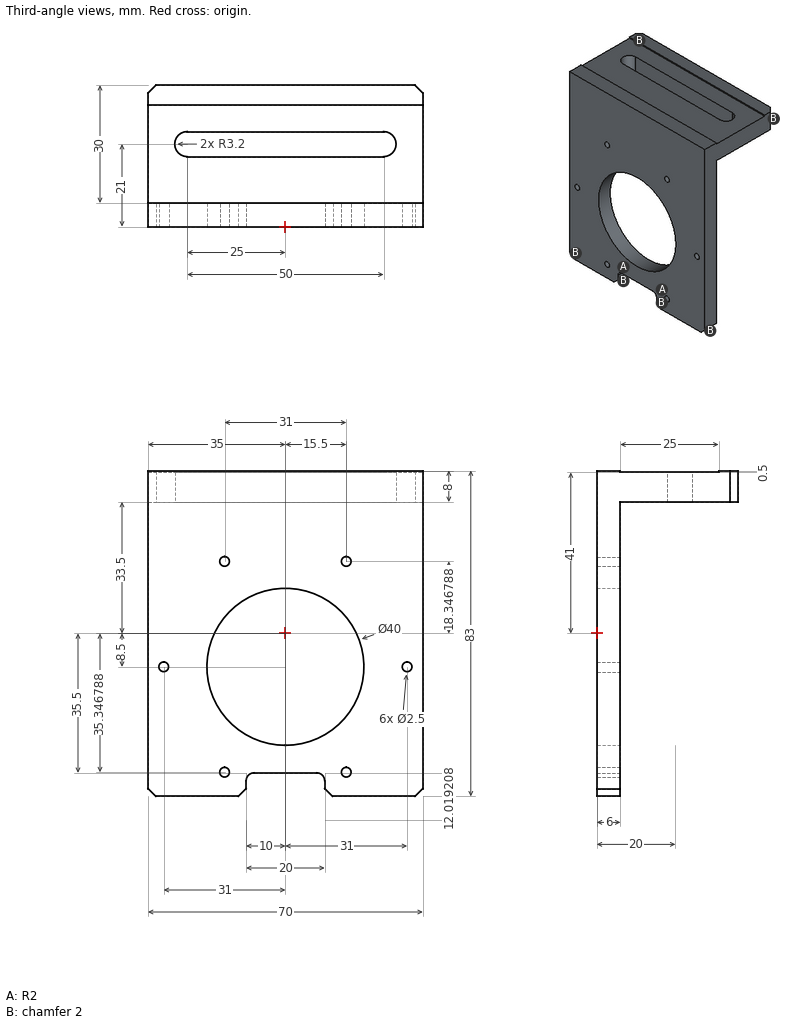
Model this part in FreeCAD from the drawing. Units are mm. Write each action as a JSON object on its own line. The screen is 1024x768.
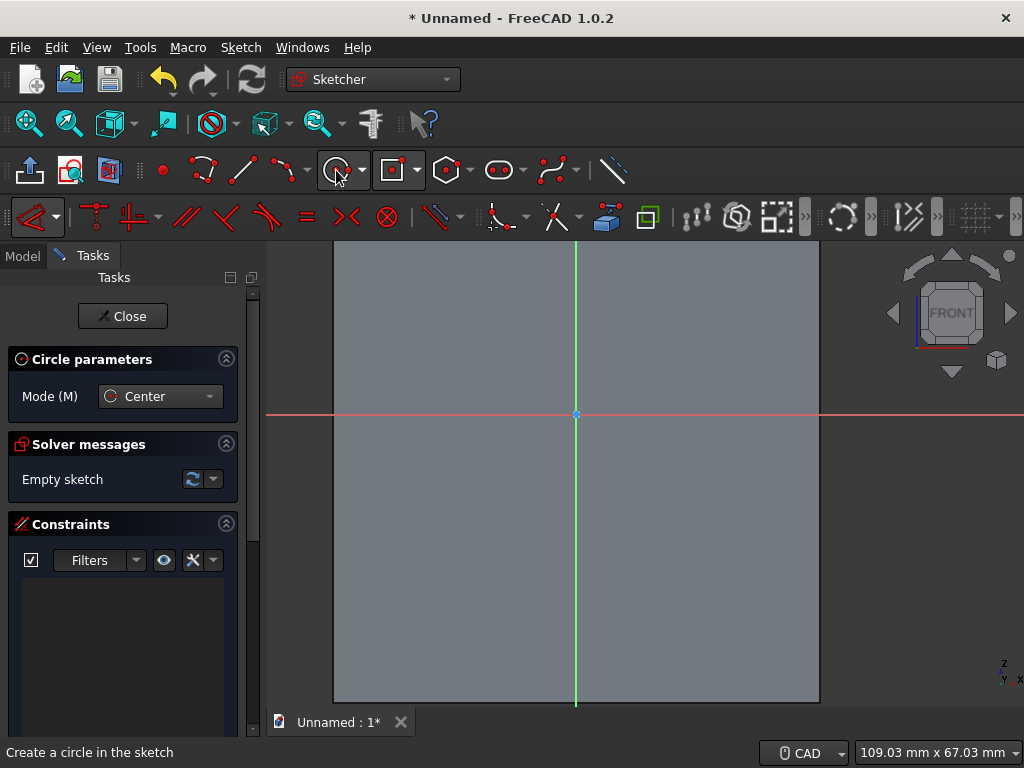
{"action": "left_click", "coordinate": [576, 474]}
{"action": "mouse_move", "coordinate": [675, 375]}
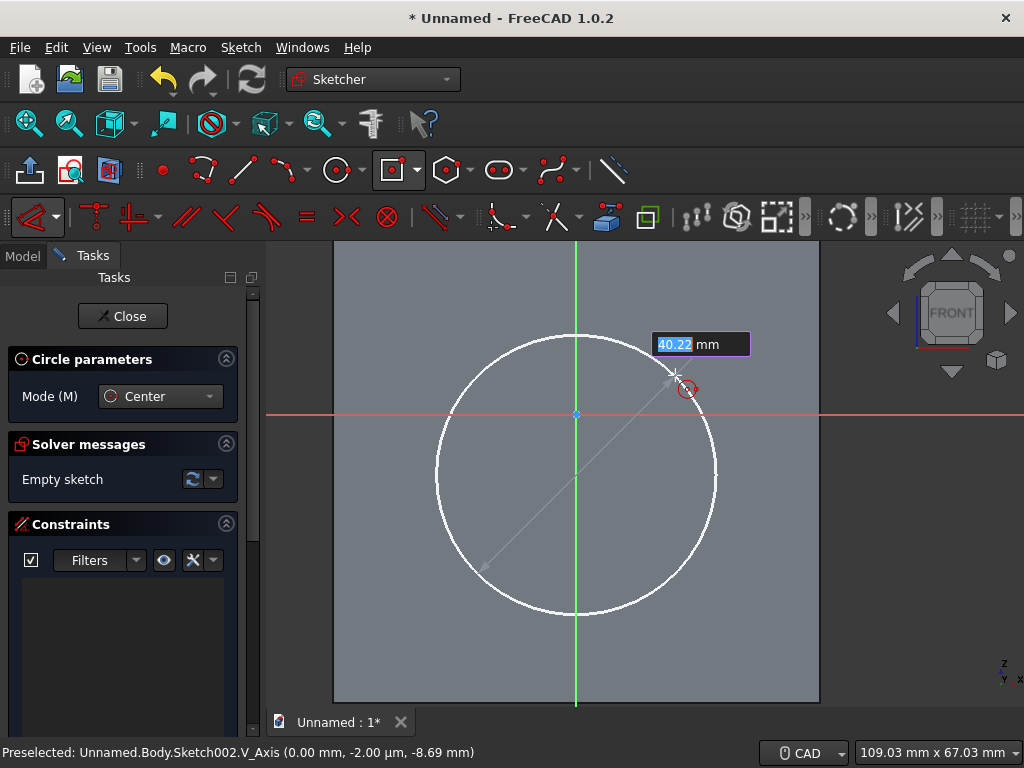
{"action": "type", "text": "40"}
{"action": "key", "text": "Return"}
{"action": "key", "text": "Escape"}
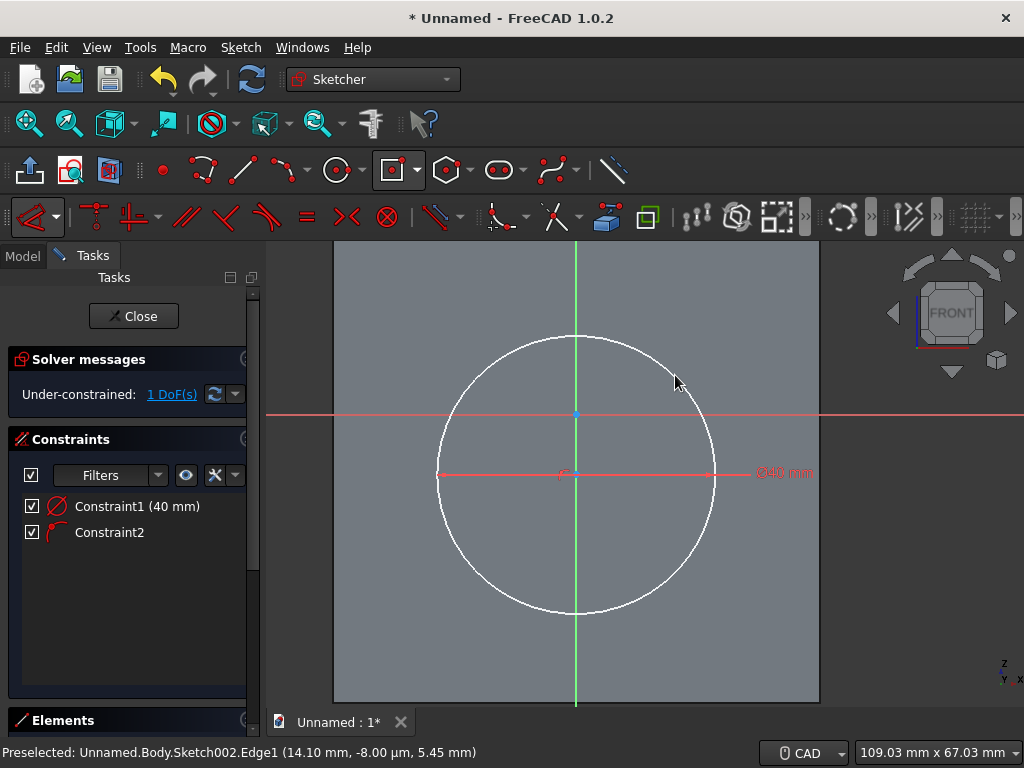
{"action": "left_click", "coordinate": [576, 475]}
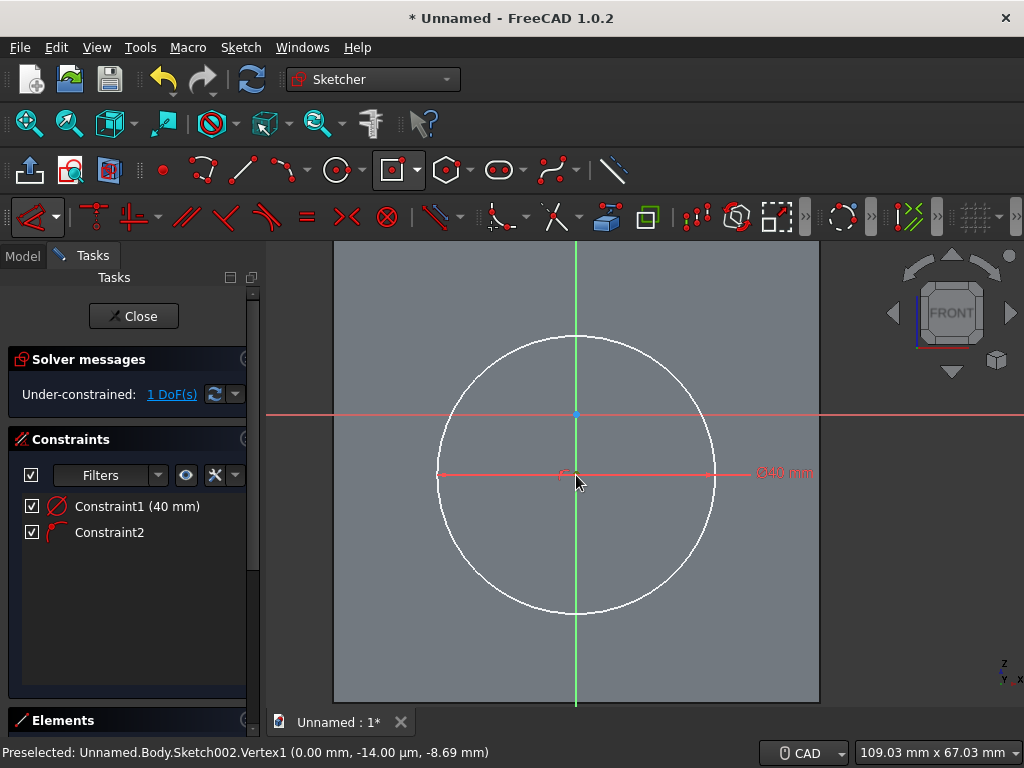
{"action": "key", "text": "i"}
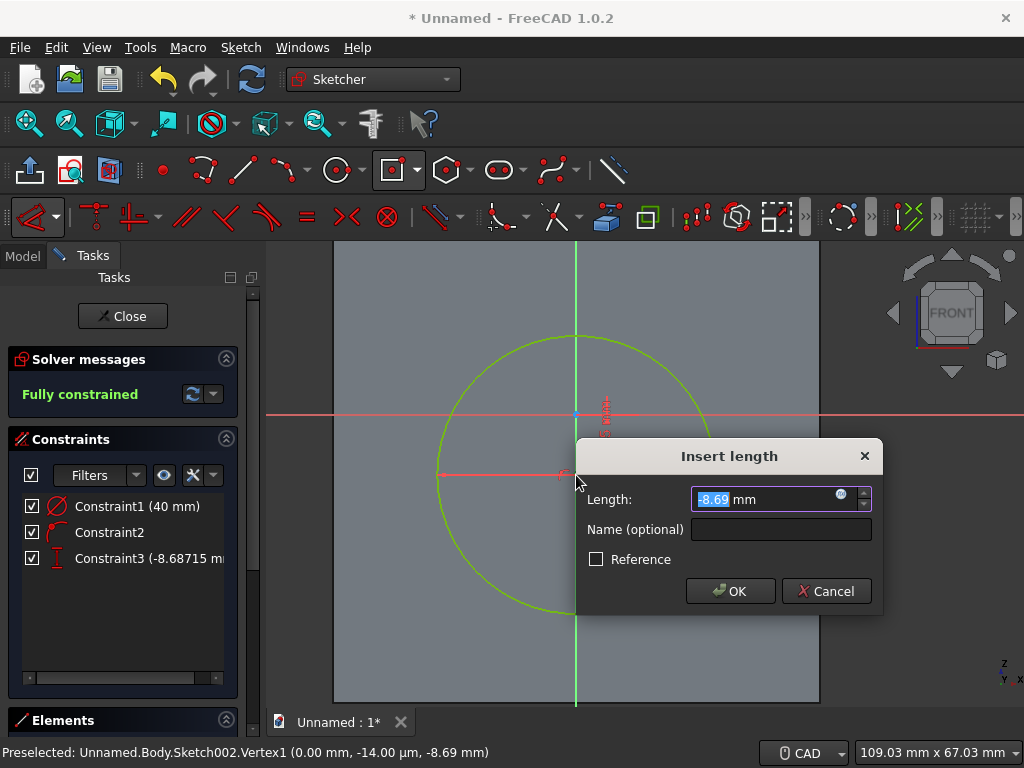
{"action": "type", "text": "-8.5"}
{"action": "key", "text": "Return"}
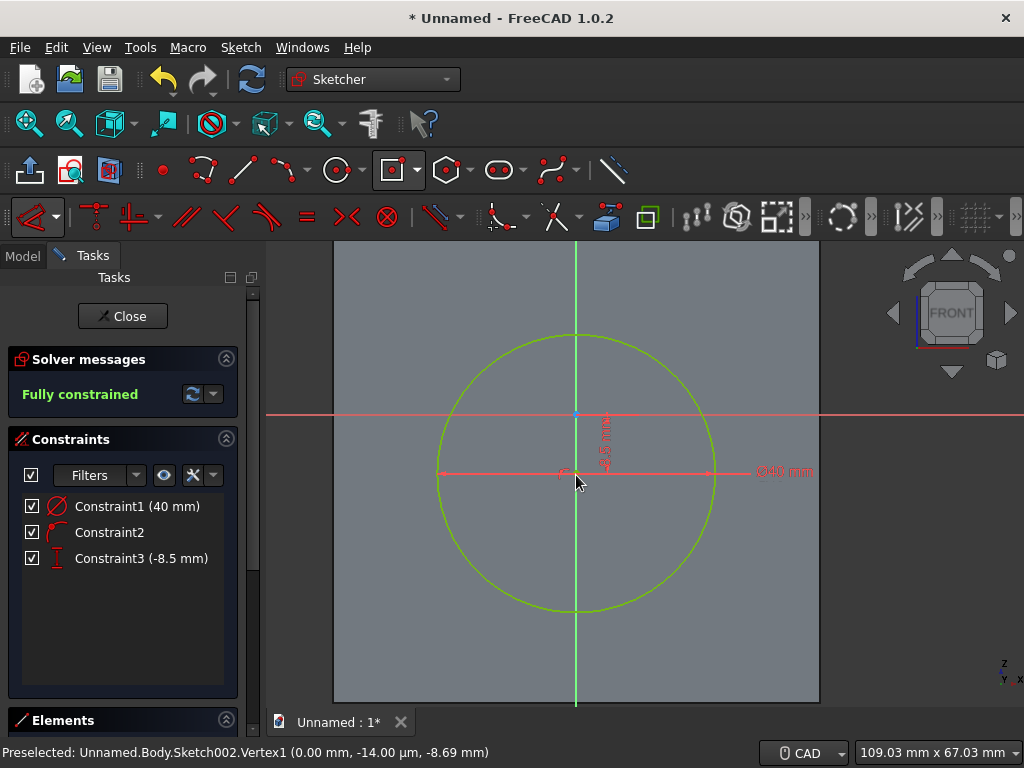
{"action": "left_click", "coordinate": [123, 316]}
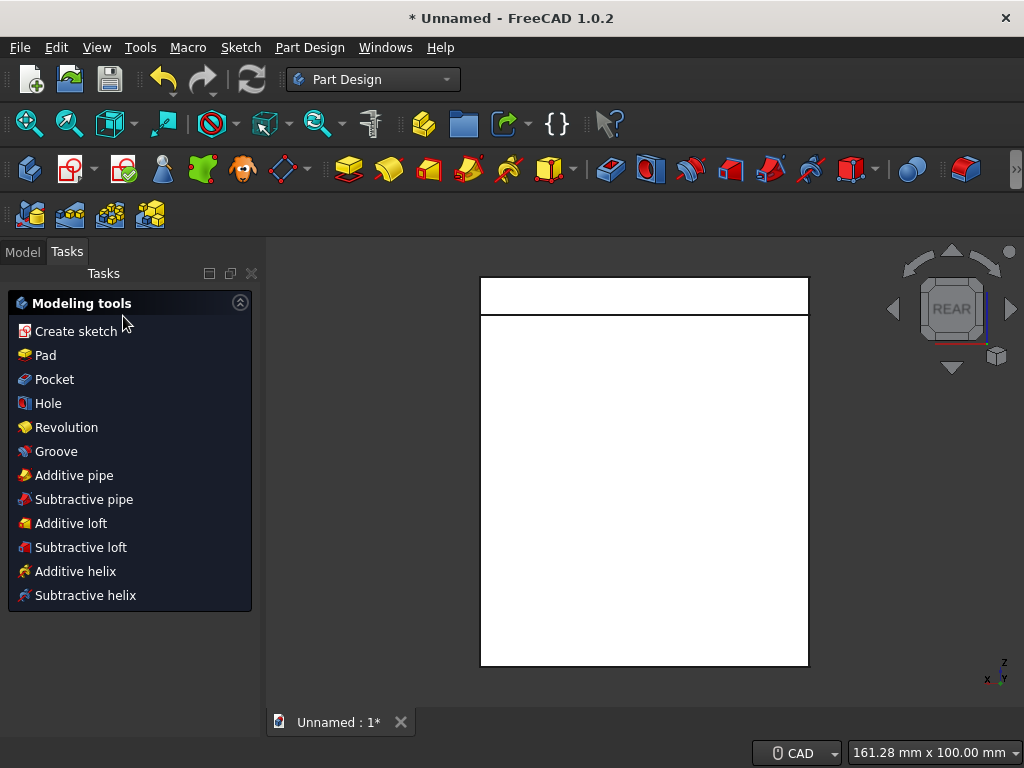
{"action": "left_click", "coordinate": [612, 170]}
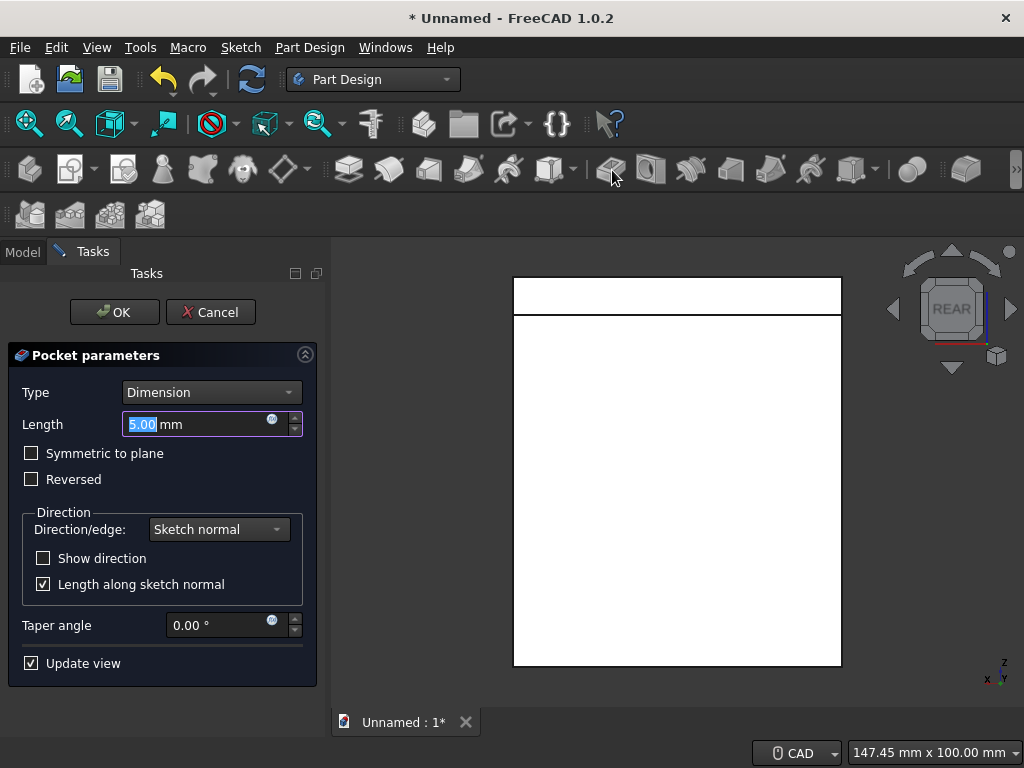
{"action": "type", "text": "20"}
{"action": "key", "text": "Tab"}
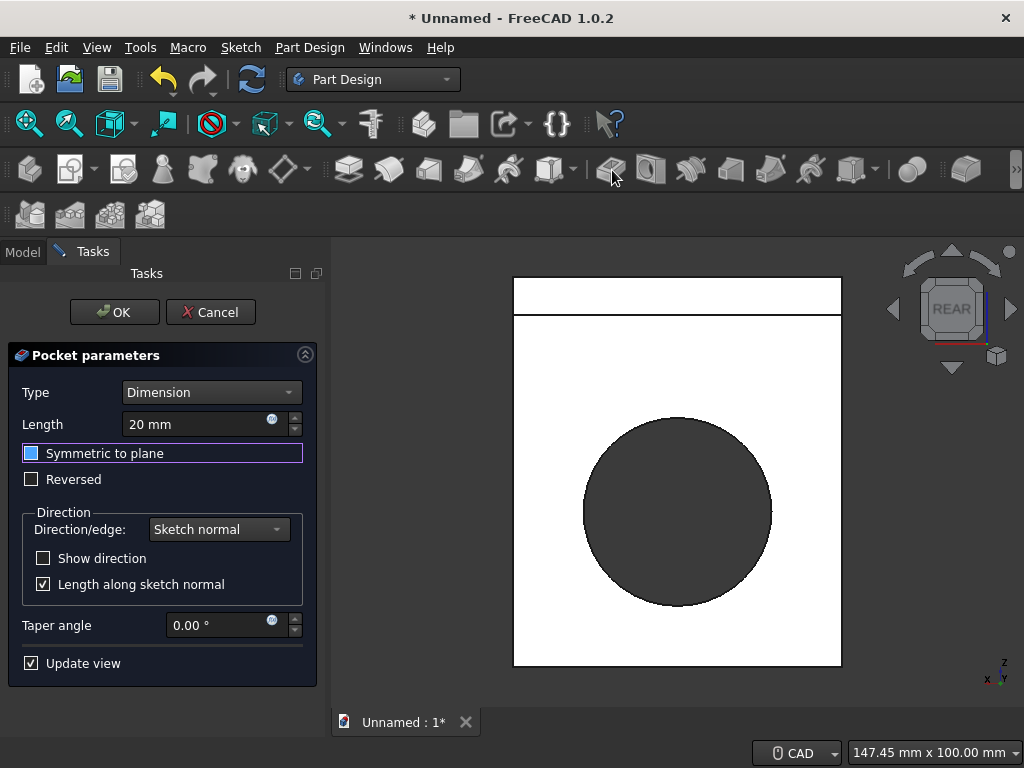
{"action": "left_click", "coordinate": [115, 312]}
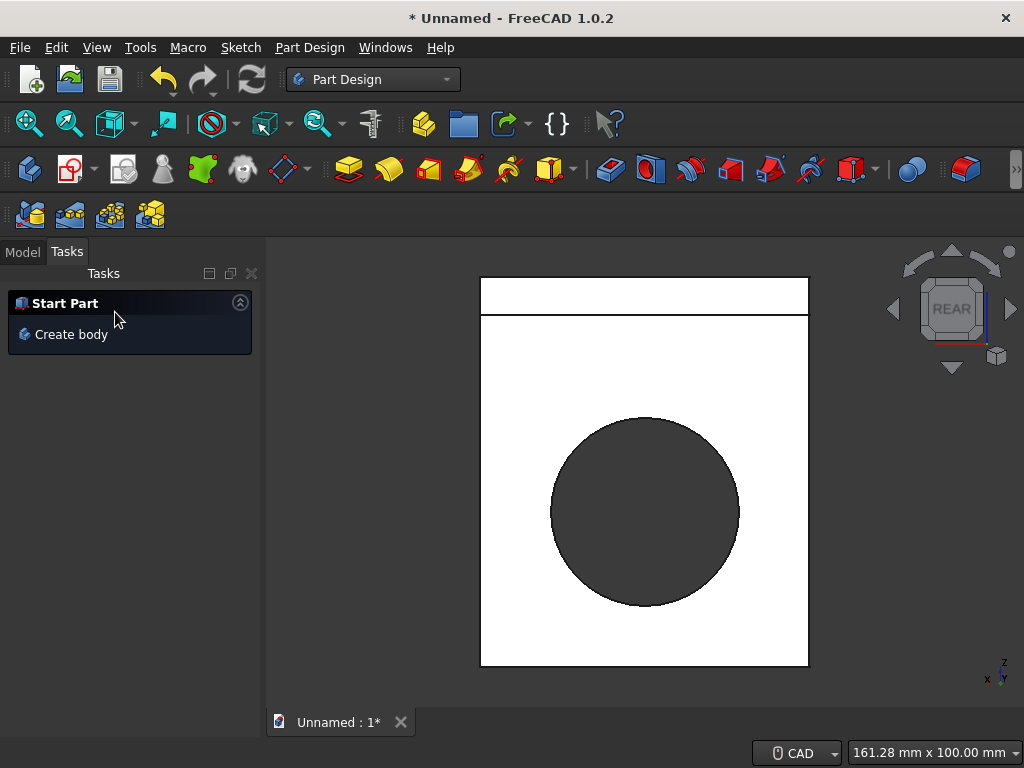
{"action": "left_click", "coordinate": [739, 389]}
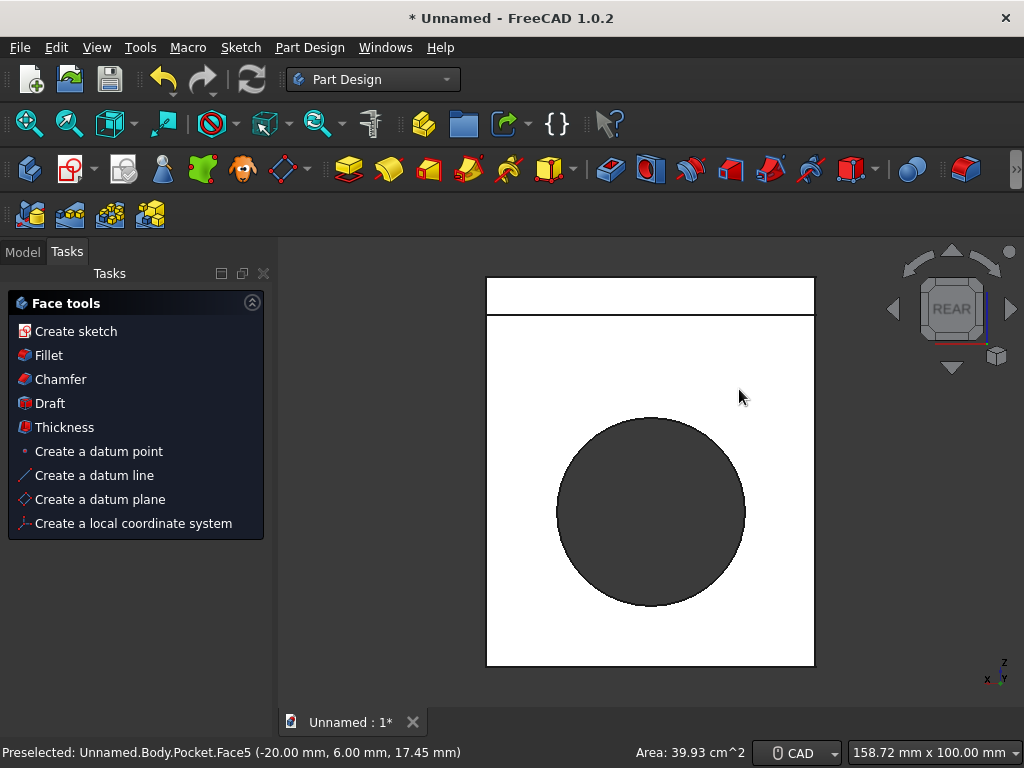
{"action": "left_click", "coordinate": [70, 170]}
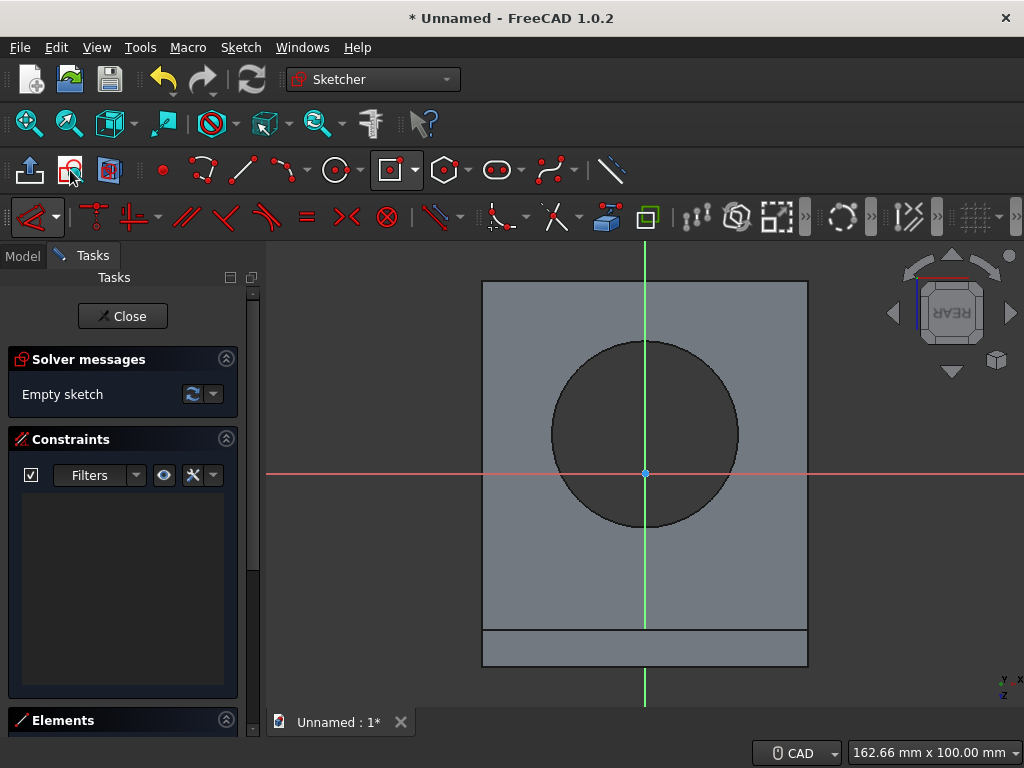
{"action": "left_click", "coordinate": [110, 170]}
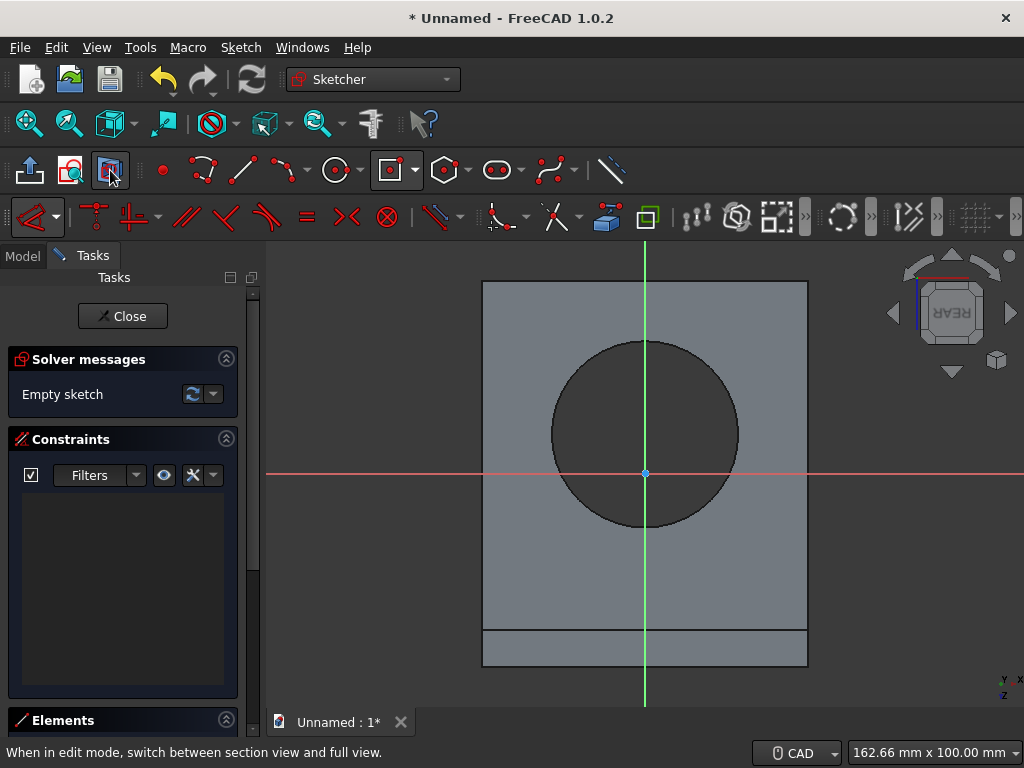
{"action": "scroll", "coordinate": [294, 679], "scroll_direction": "down", "scroll_amount": 1}